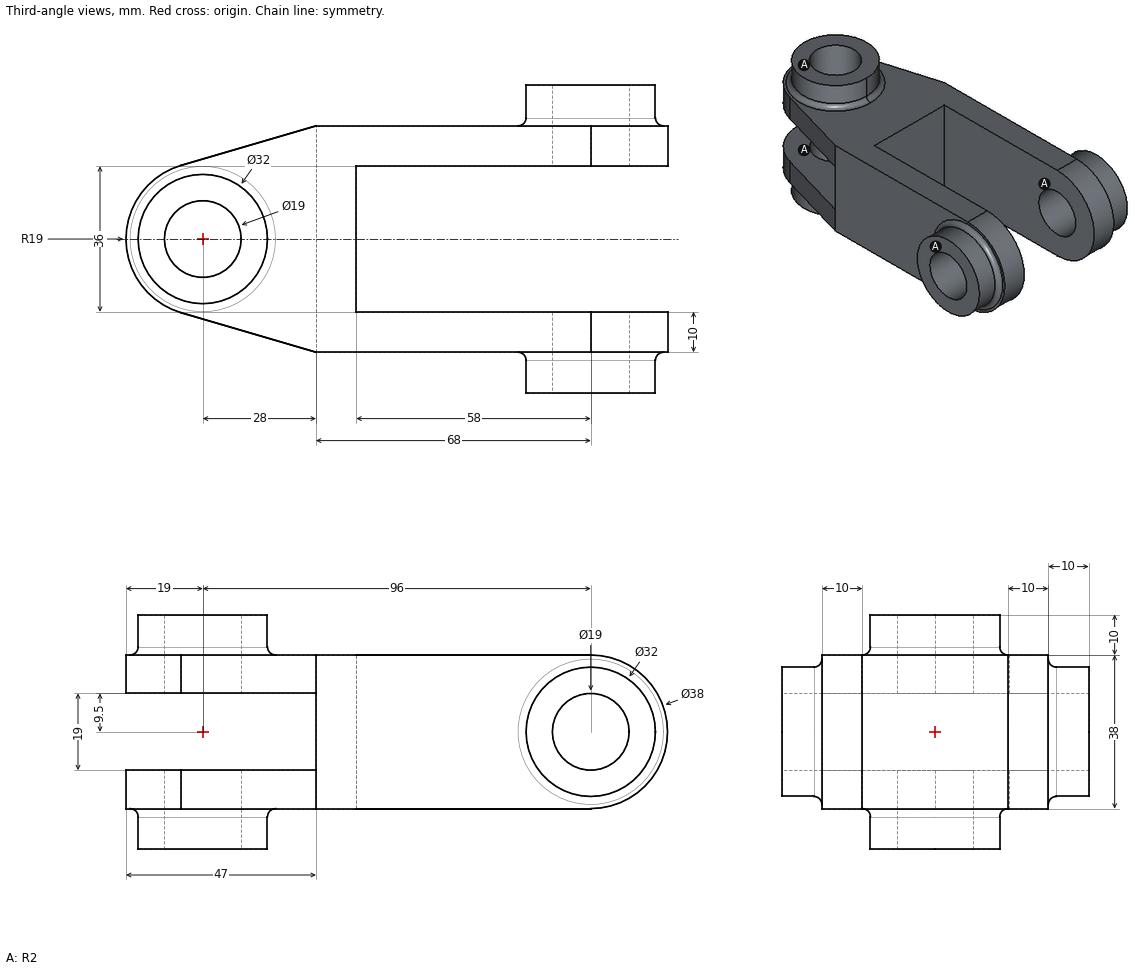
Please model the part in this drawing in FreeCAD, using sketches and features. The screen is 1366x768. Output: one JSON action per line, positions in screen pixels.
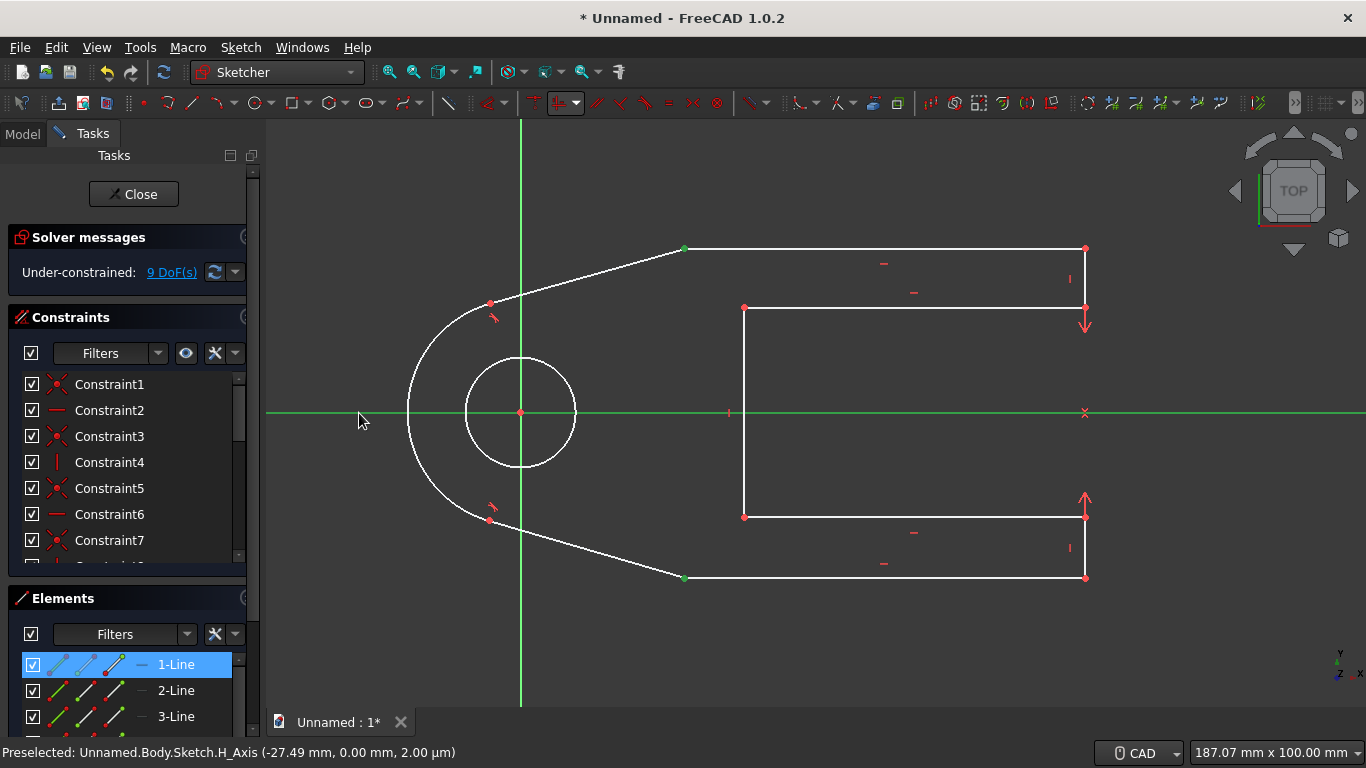
{"action": "left_click", "coordinate": [694, 104]}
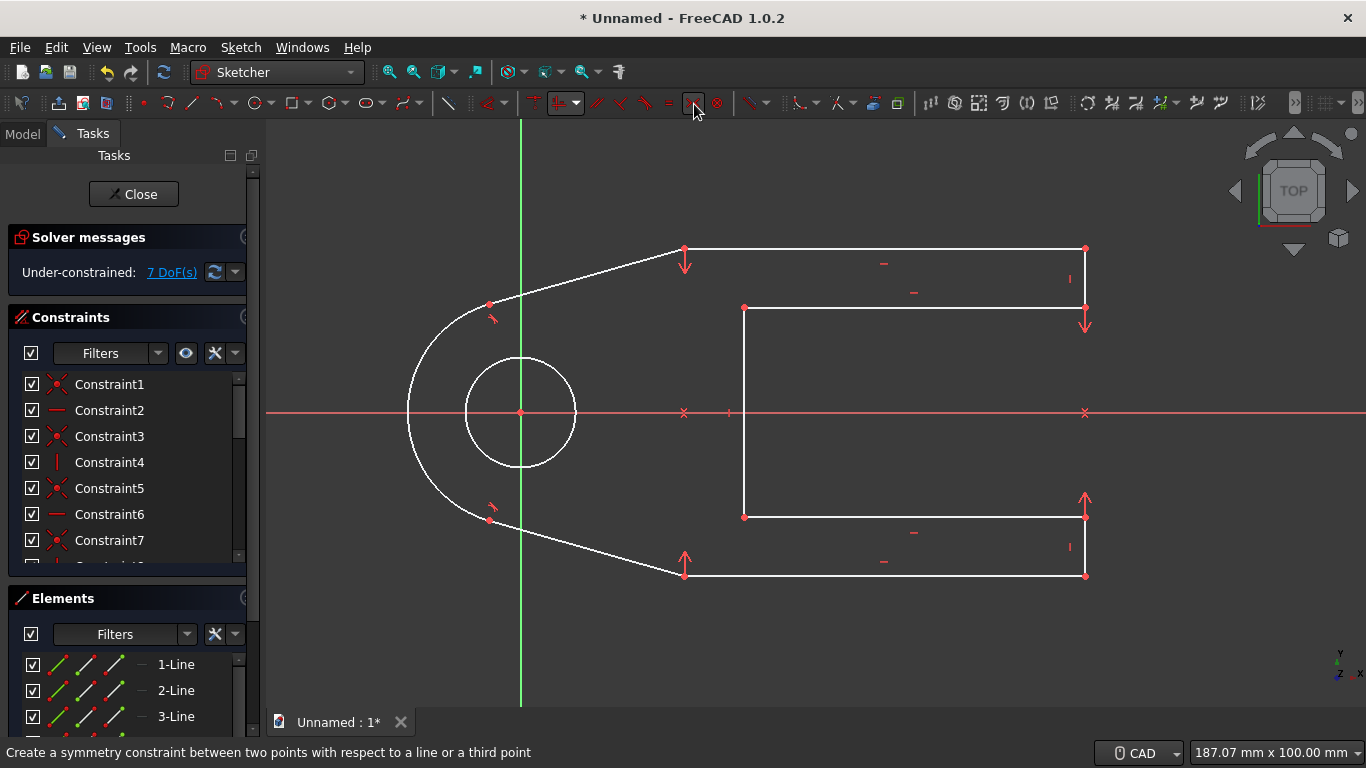
{"action": "left_click", "coordinate": [488, 104]}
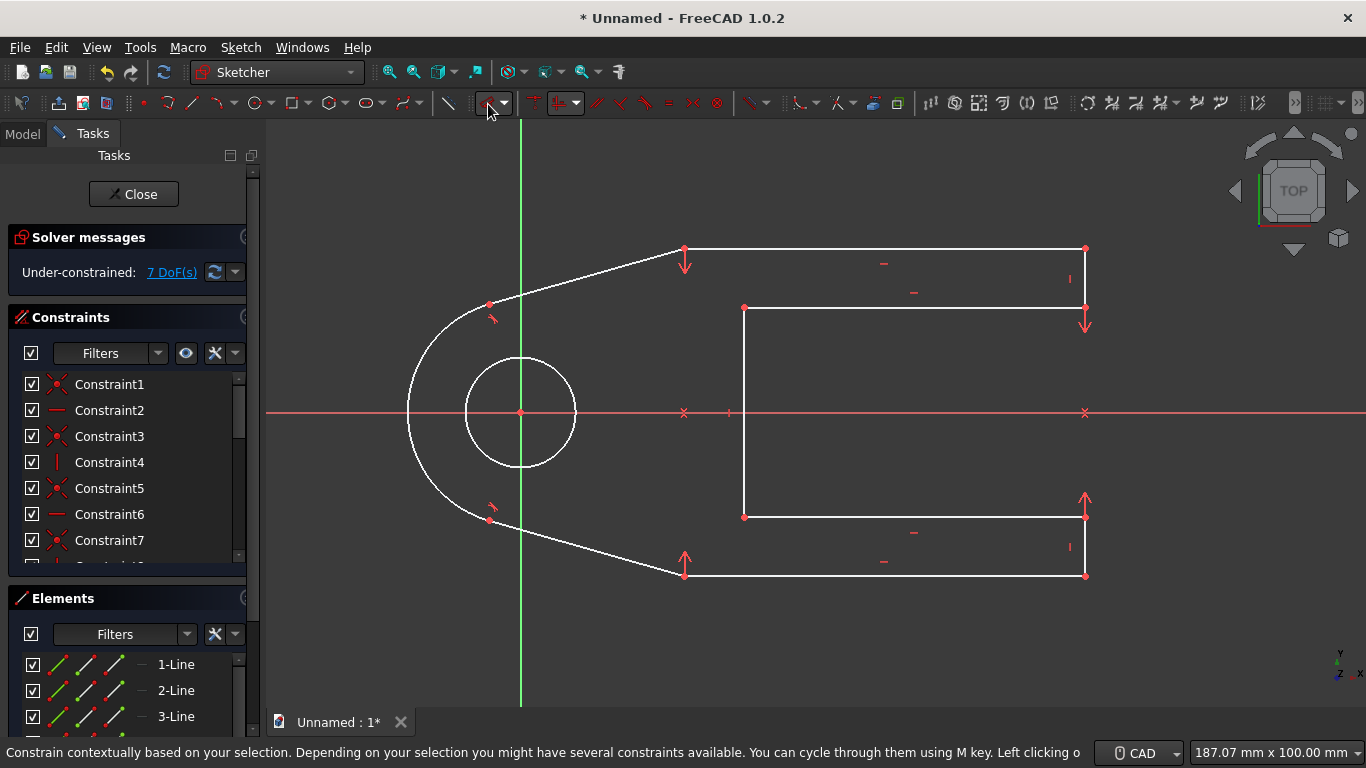
{"action": "left_click", "coordinate": [423, 357]}
{"action": "left_click", "coordinate": [395, 341]}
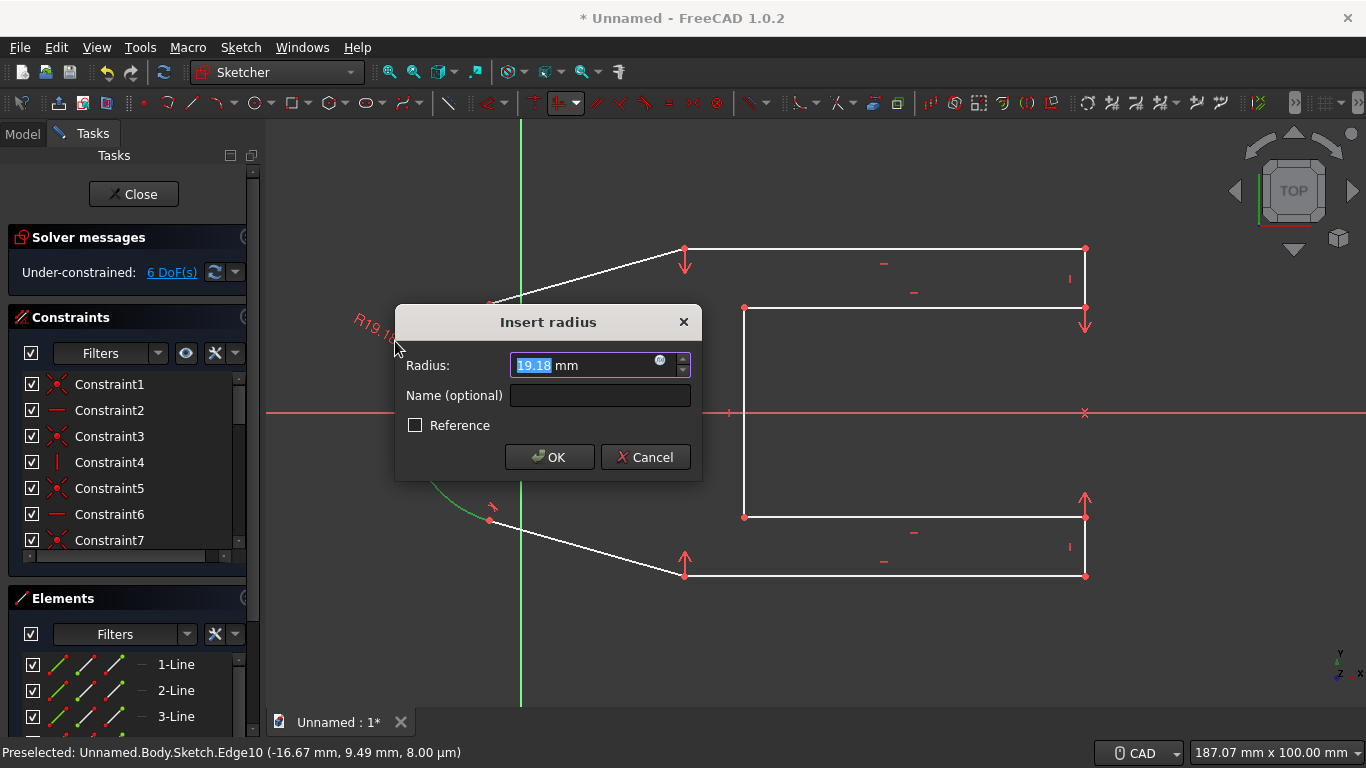
{"action": "type", "text": "19"}
{"action": "key", "text": "Return"}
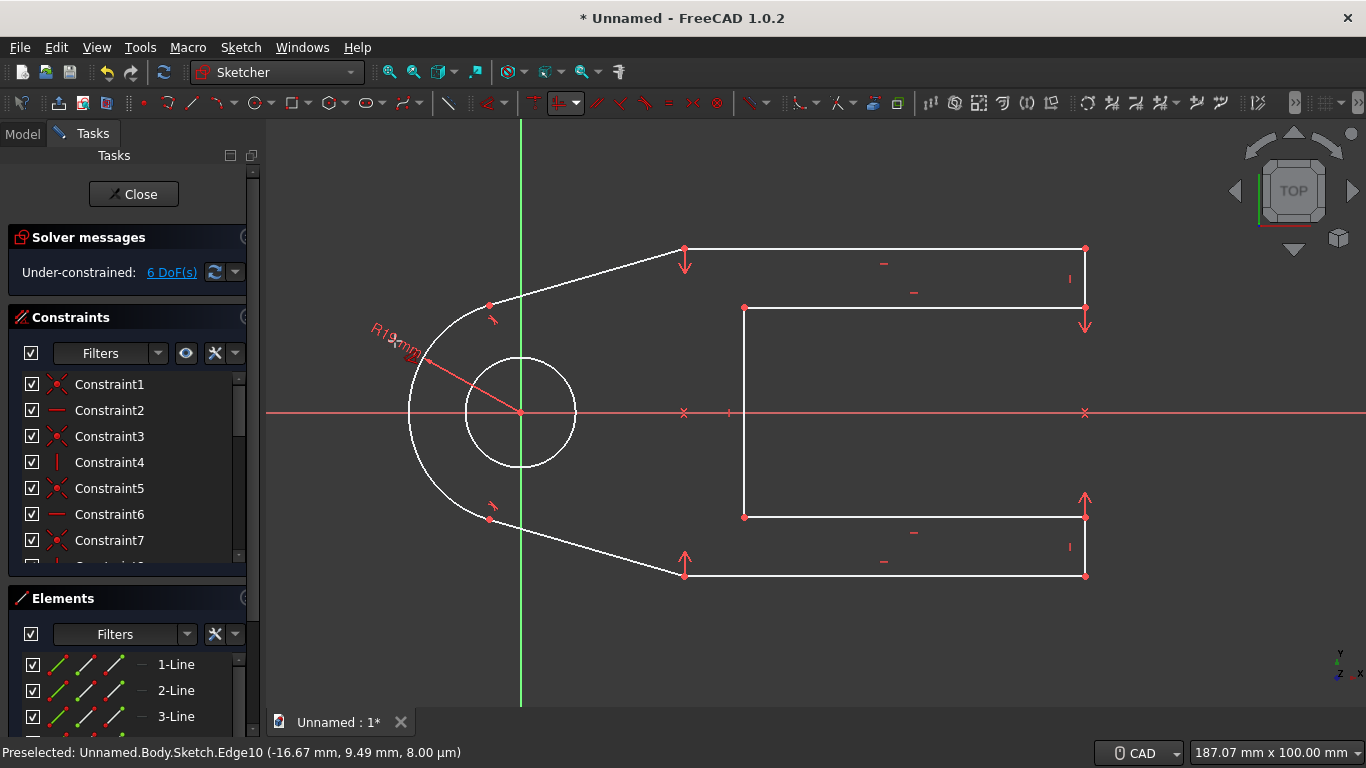
{"action": "left_click", "coordinate": [559, 373]}
{"action": "left_click", "coordinate": [581, 350]}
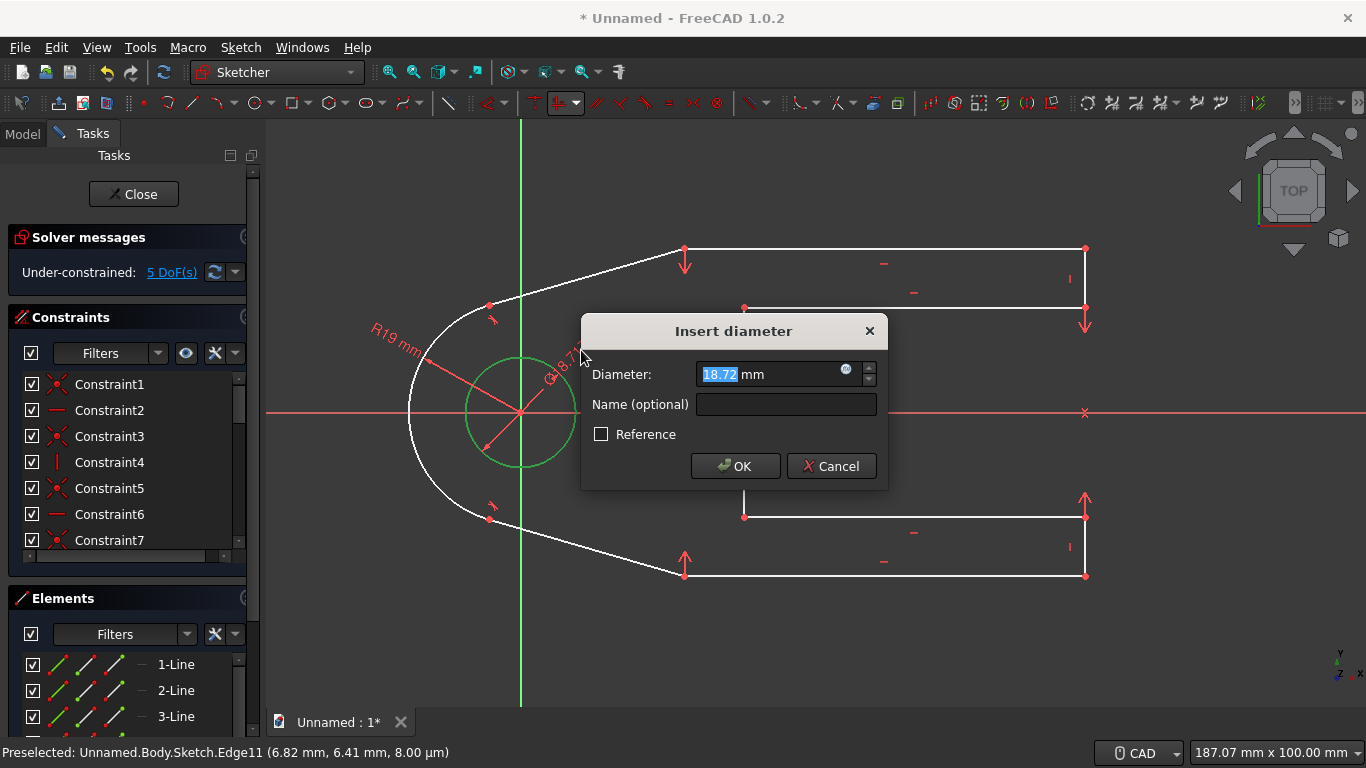
{"action": "type", "text": "19"}
{"action": "key", "text": "Return"}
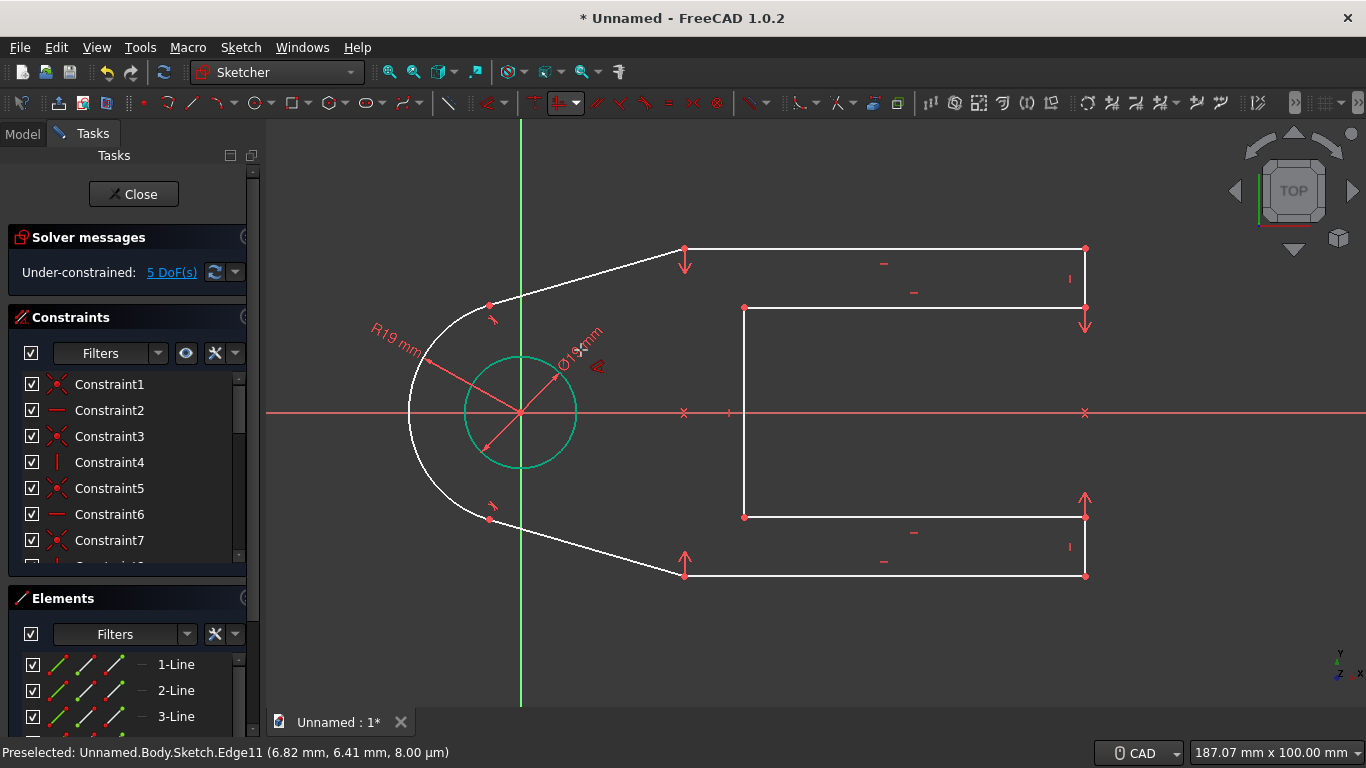
{"action": "left_click", "coordinate": [805, 576]}
{"action": "left_click", "coordinate": [885, 610]}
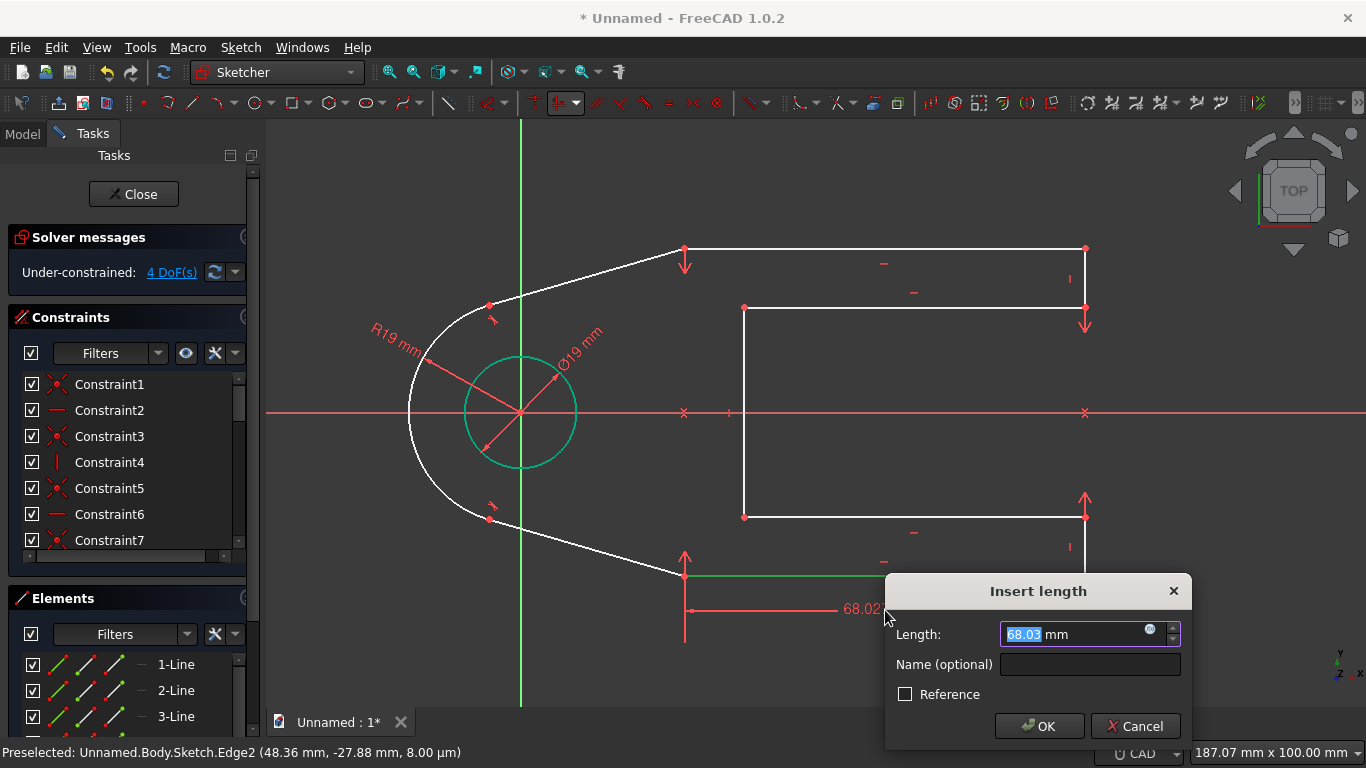
{"action": "type", "text": "68"}
{"action": "key", "text": "Return"}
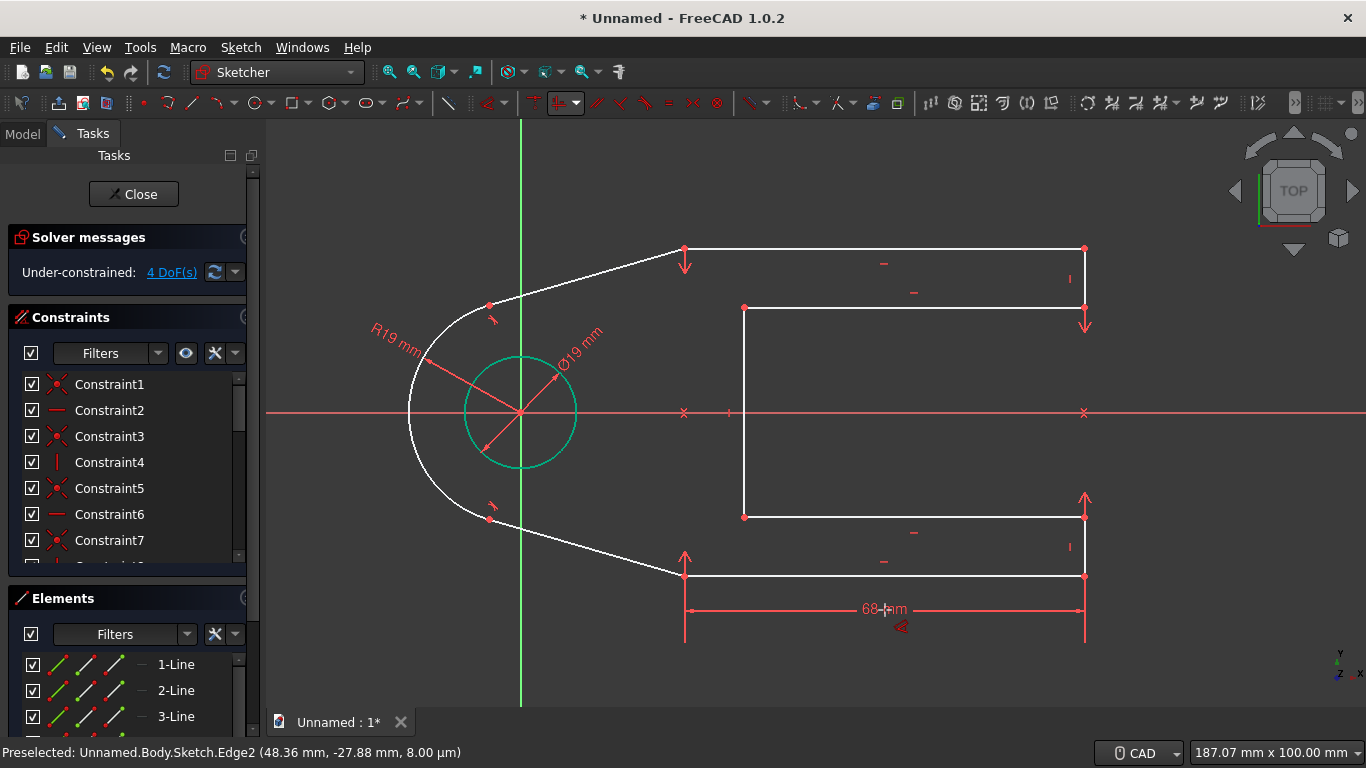
{"action": "left_click", "coordinate": [1085, 559]}
{"action": "left_click", "coordinate": [1119, 547]}